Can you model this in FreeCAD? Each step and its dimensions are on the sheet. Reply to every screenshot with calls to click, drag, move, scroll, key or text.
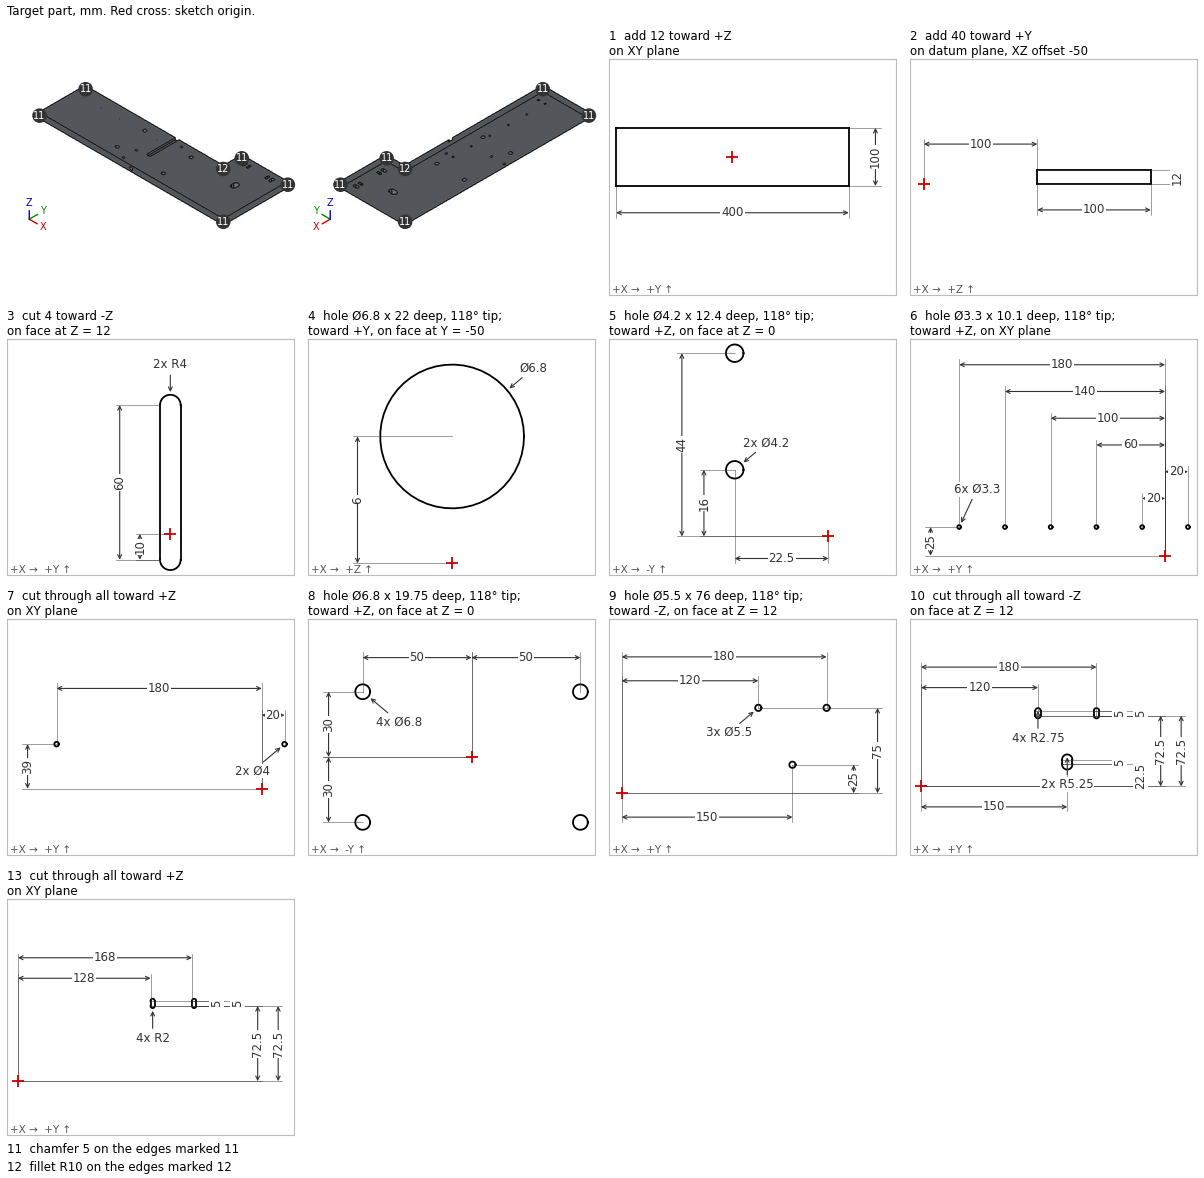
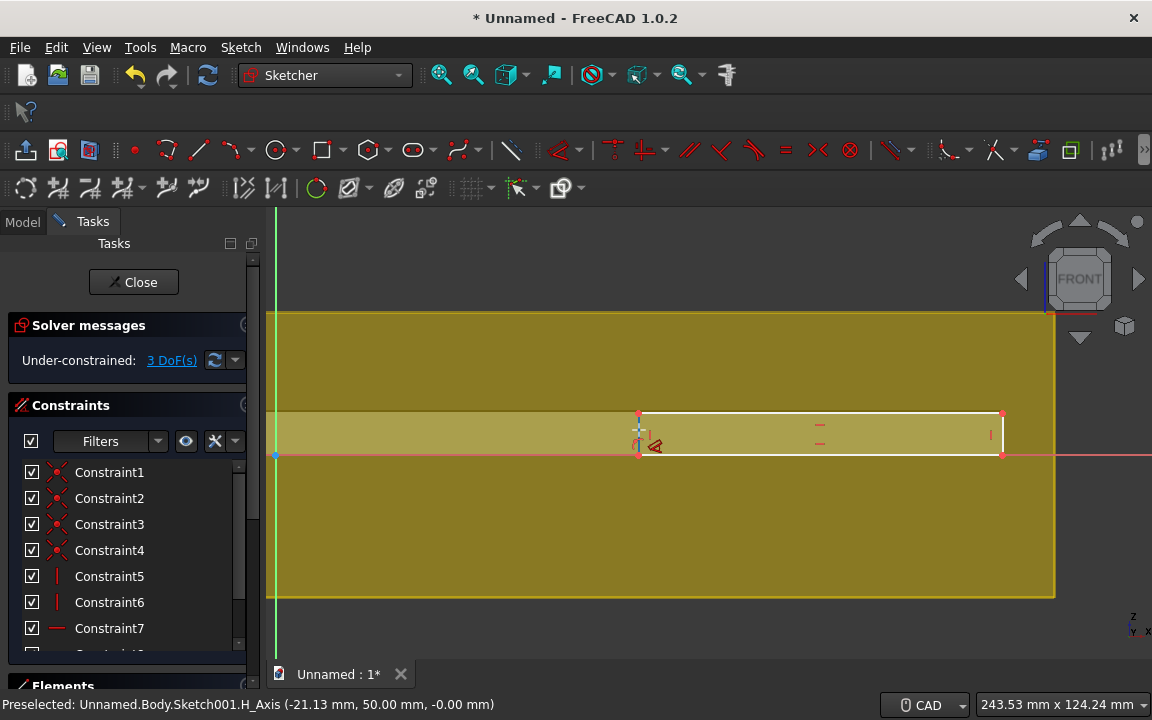
click(639, 430)
click(605, 434)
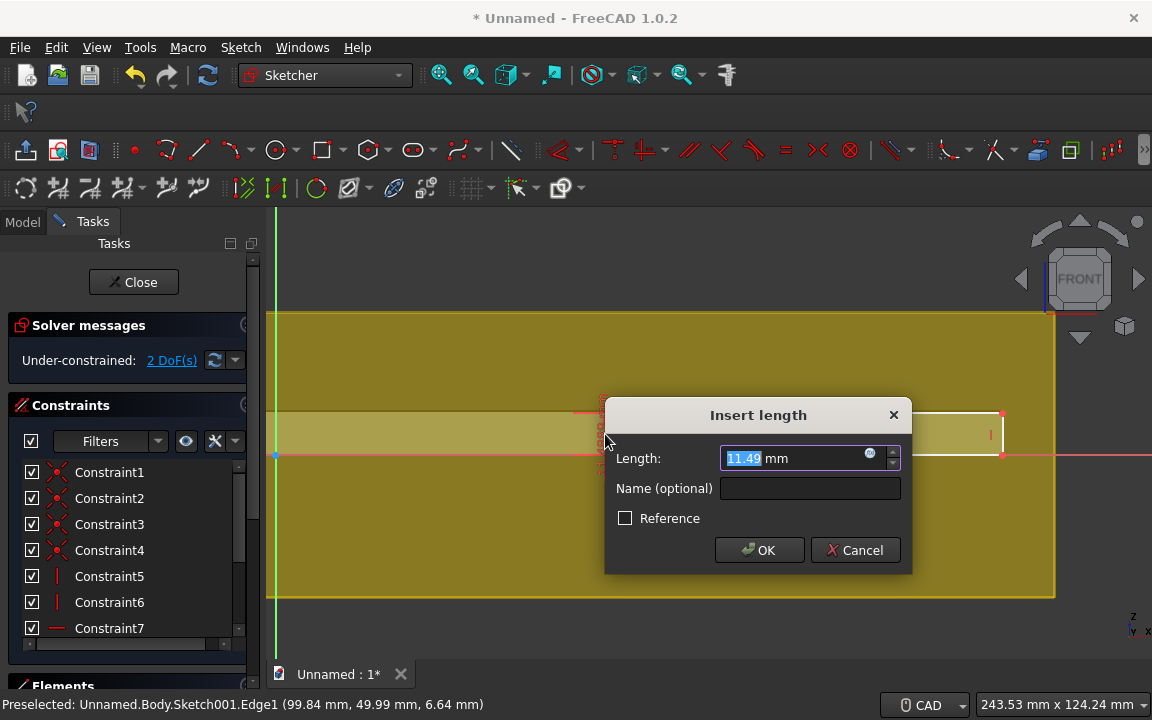
text(12)
key(Return)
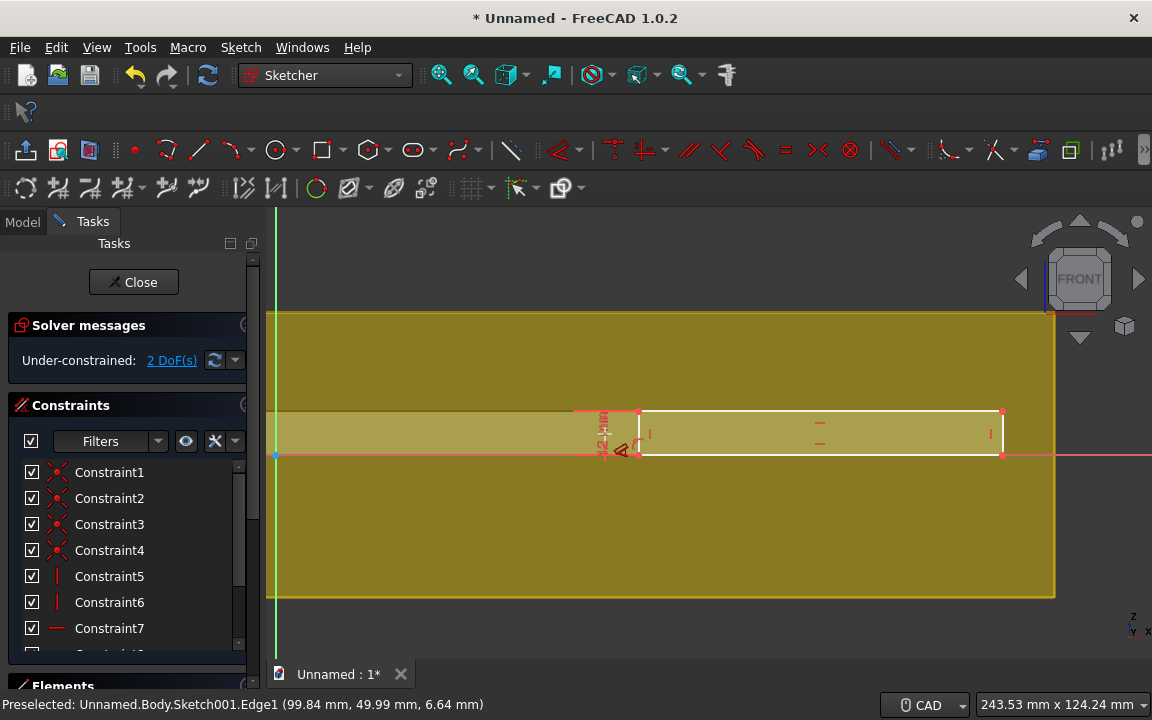
click(748, 455)
click(813, 489)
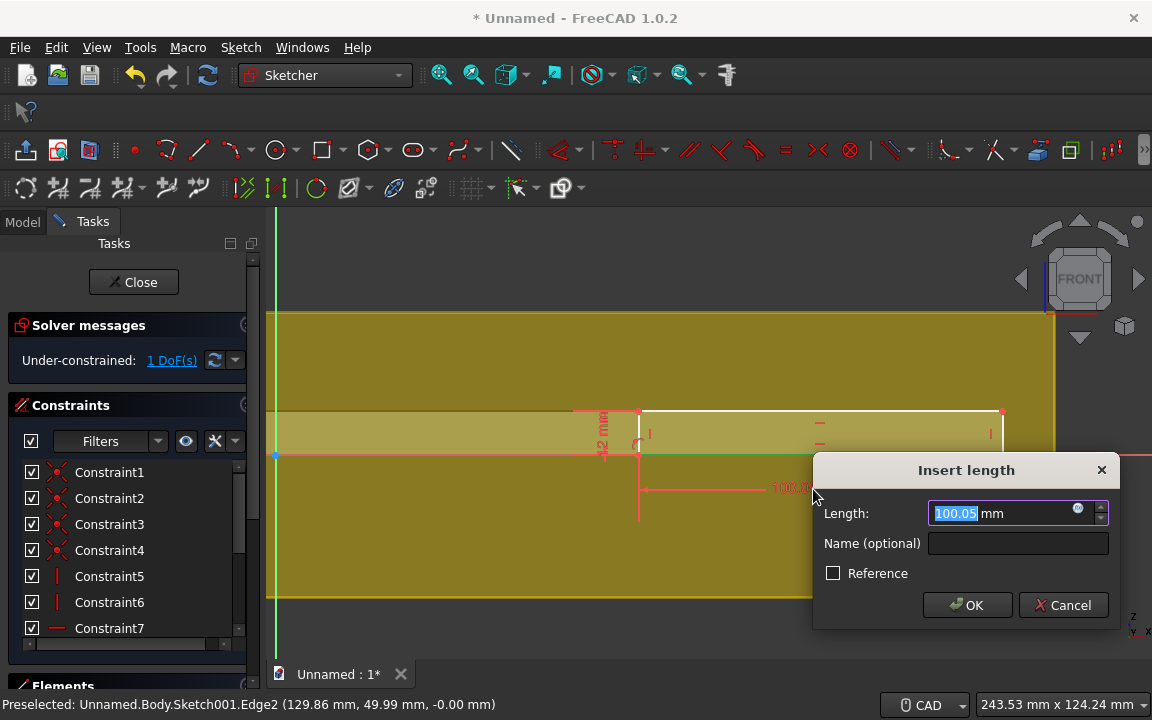
text(100)
key(Return)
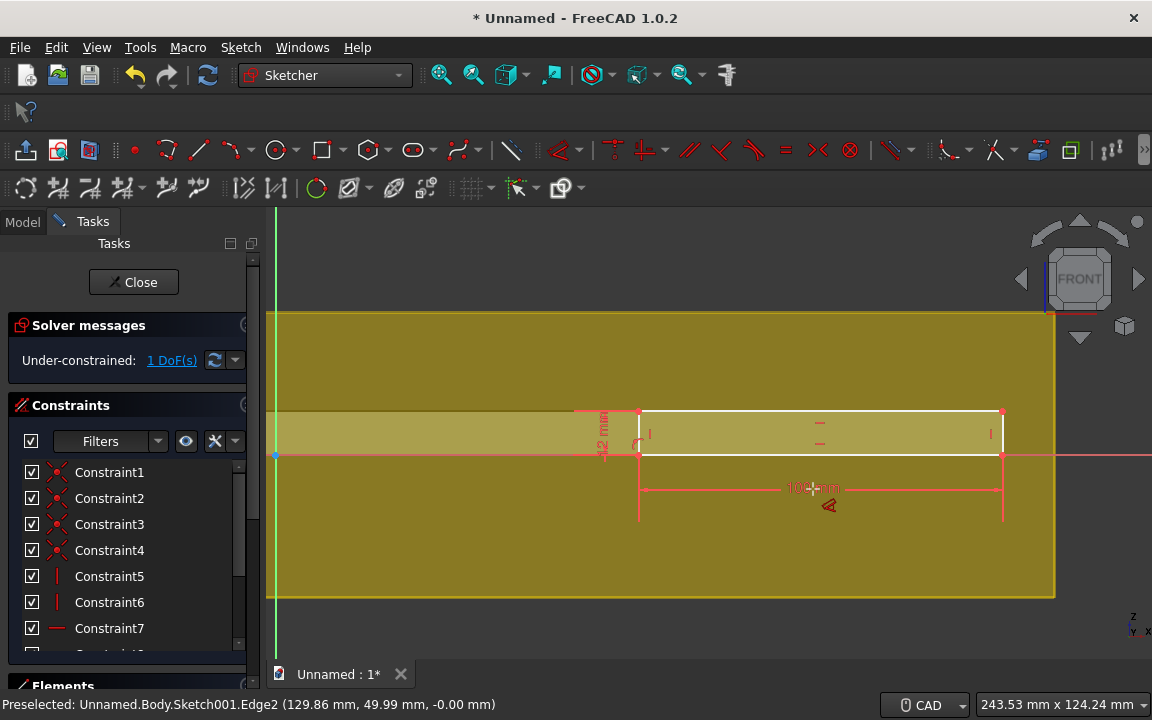
click(639, 411)
click(466, 489)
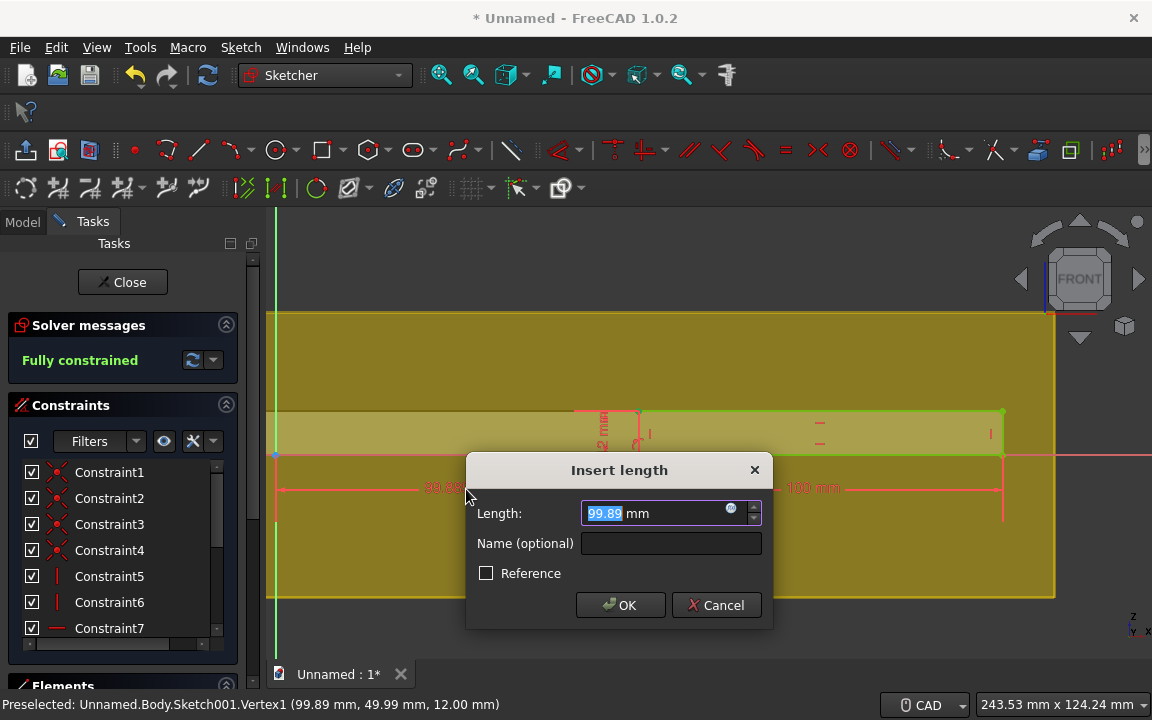
text(100)
key(Return)
key(Escape)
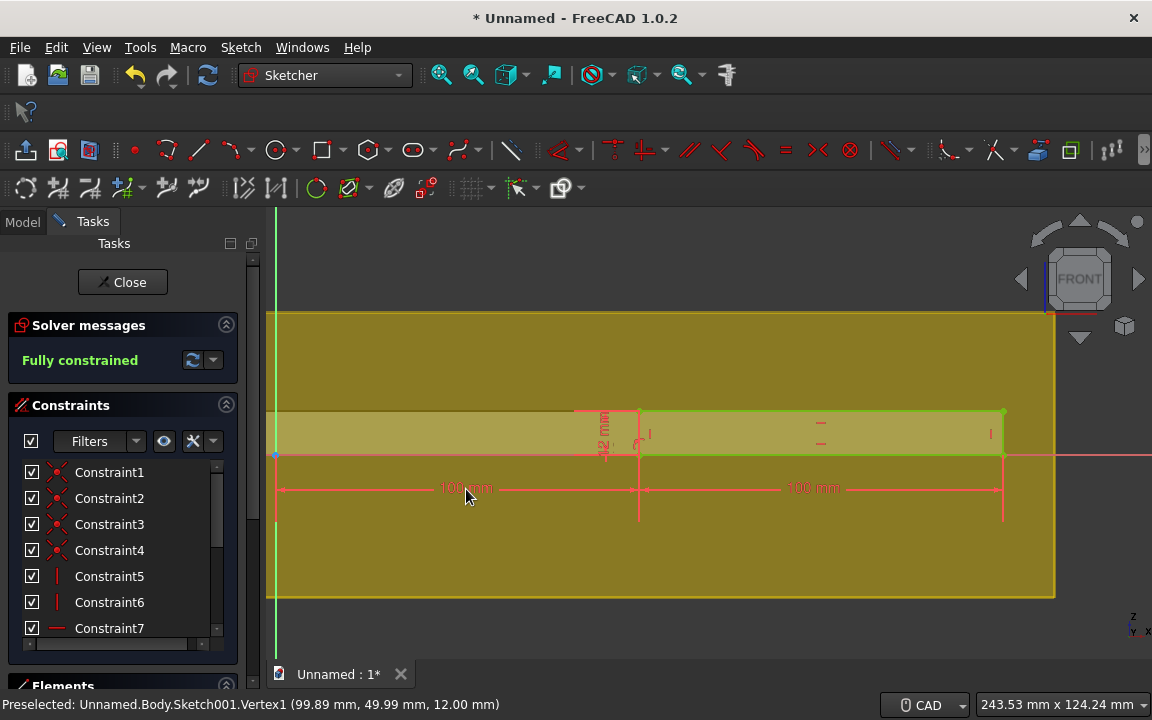
click(123, 282)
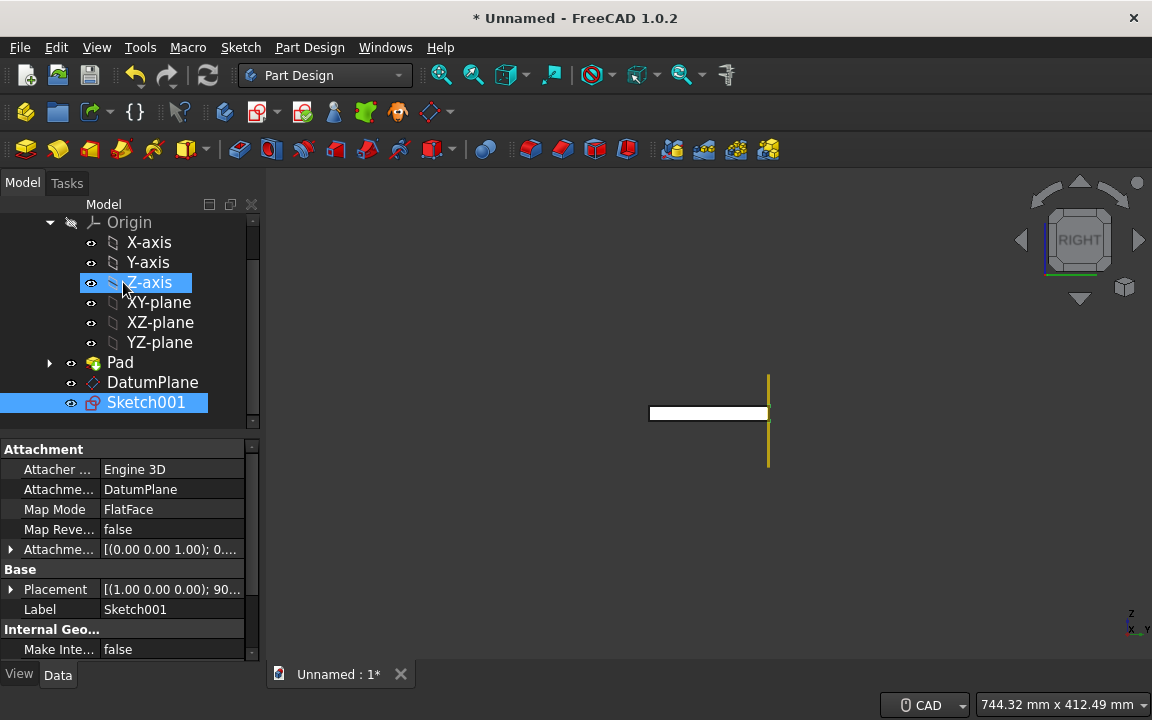
click(26, 150)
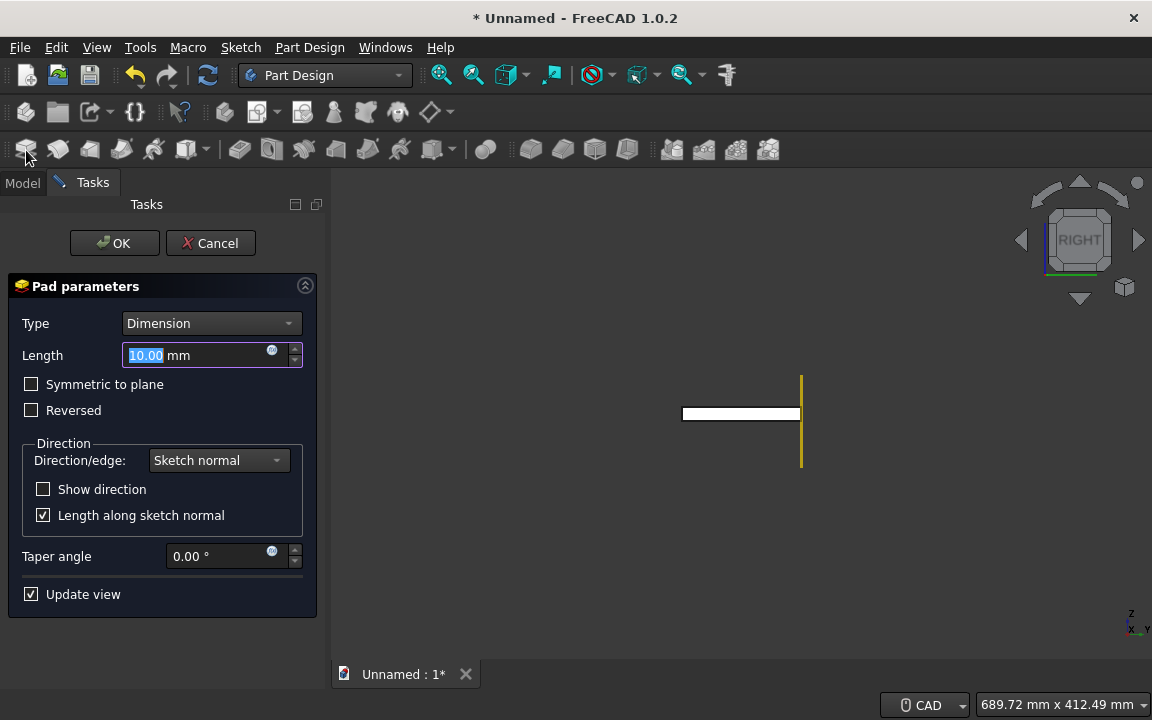
text(40)
key(Tab)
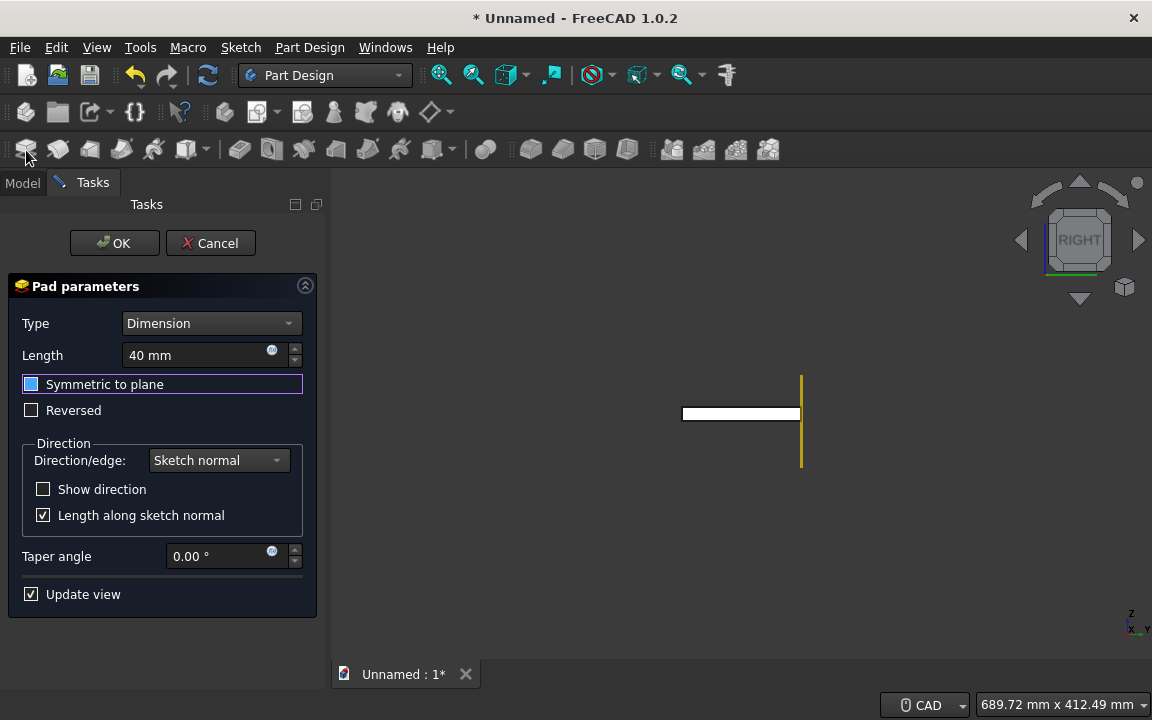
click(30, 410)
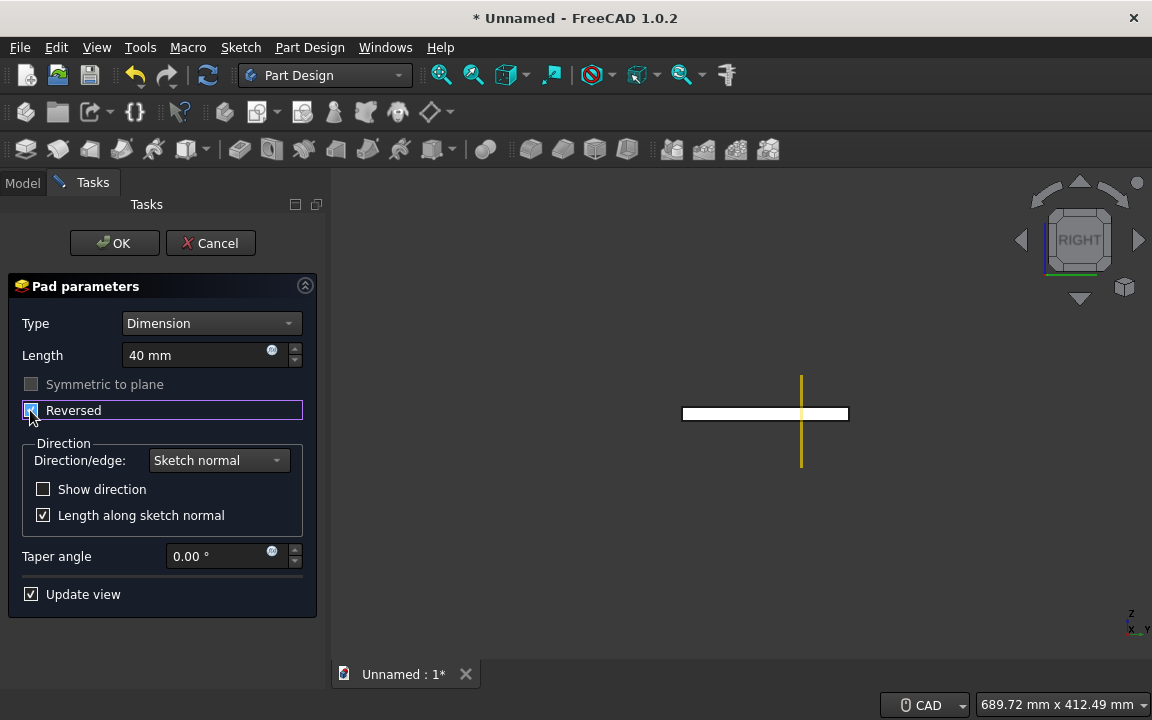
click(115, 243)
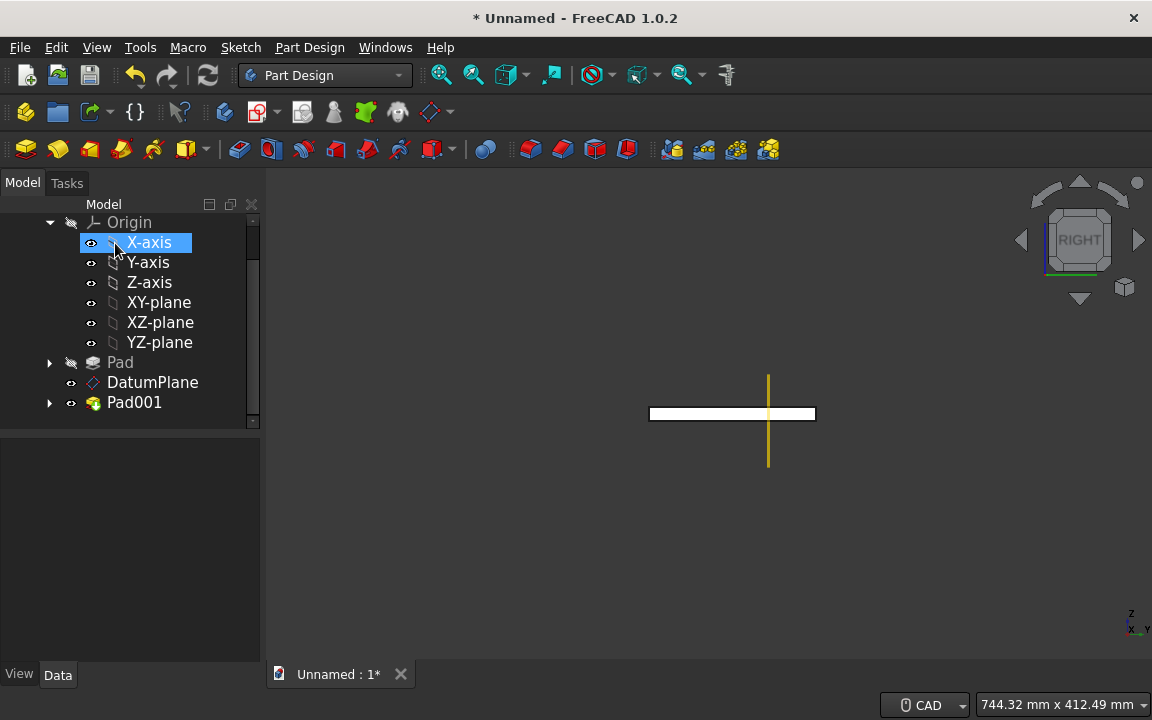
click(116, 383)
key(space)